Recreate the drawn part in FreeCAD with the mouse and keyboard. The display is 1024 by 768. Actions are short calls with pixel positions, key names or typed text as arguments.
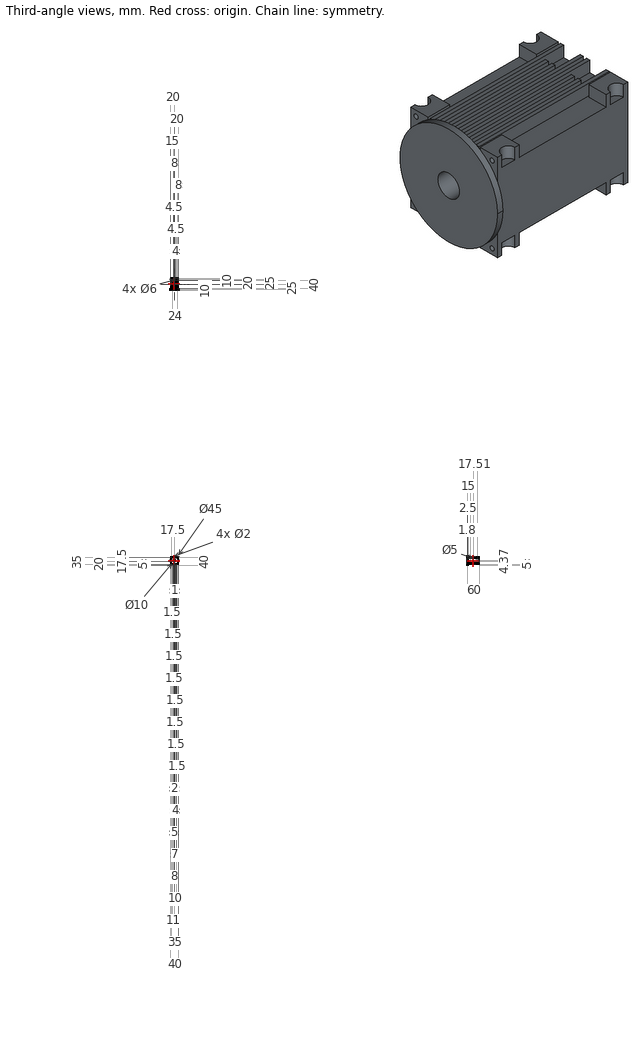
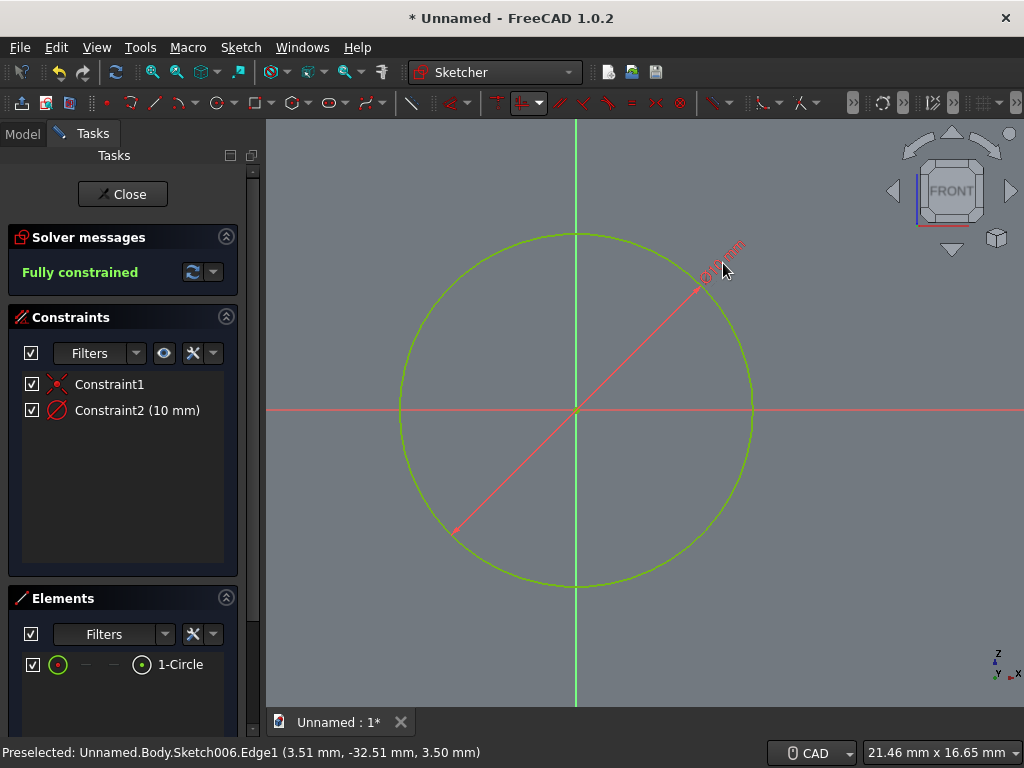
click(123, 194)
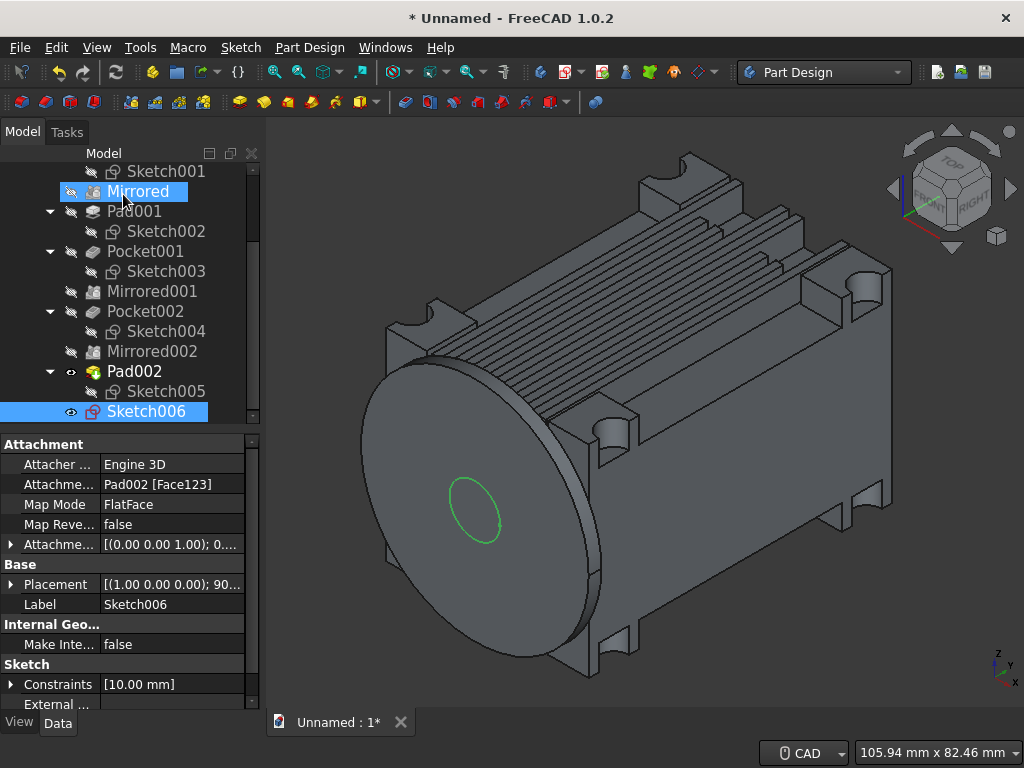
click(406, 102)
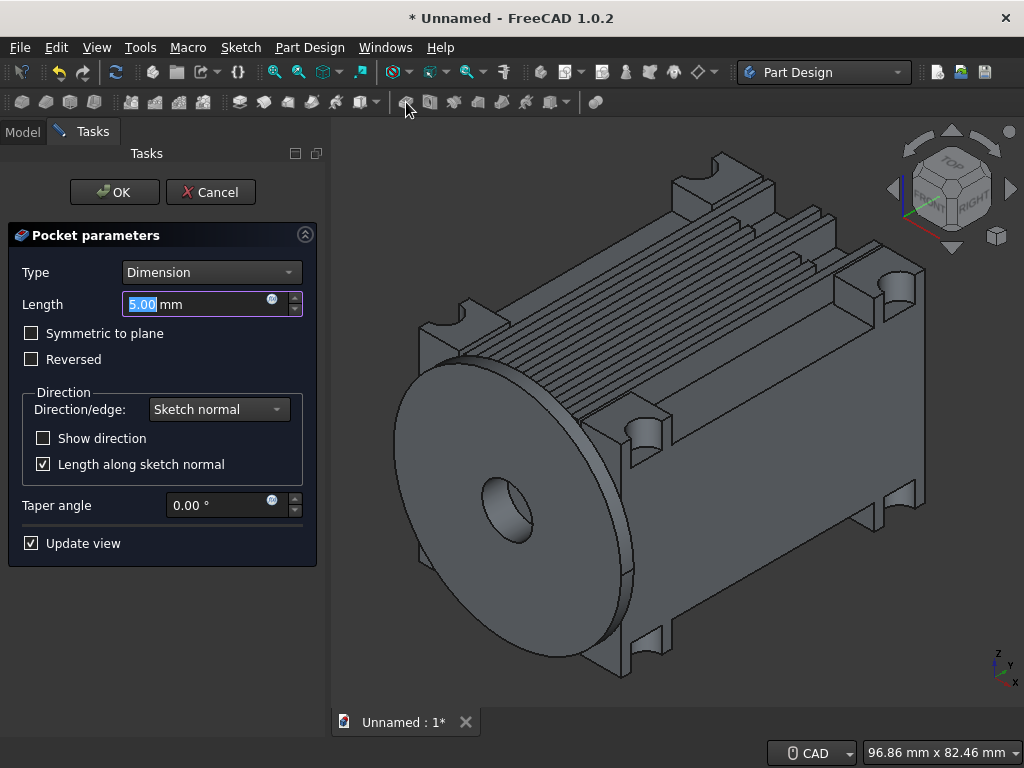
text(15)
key(Tab)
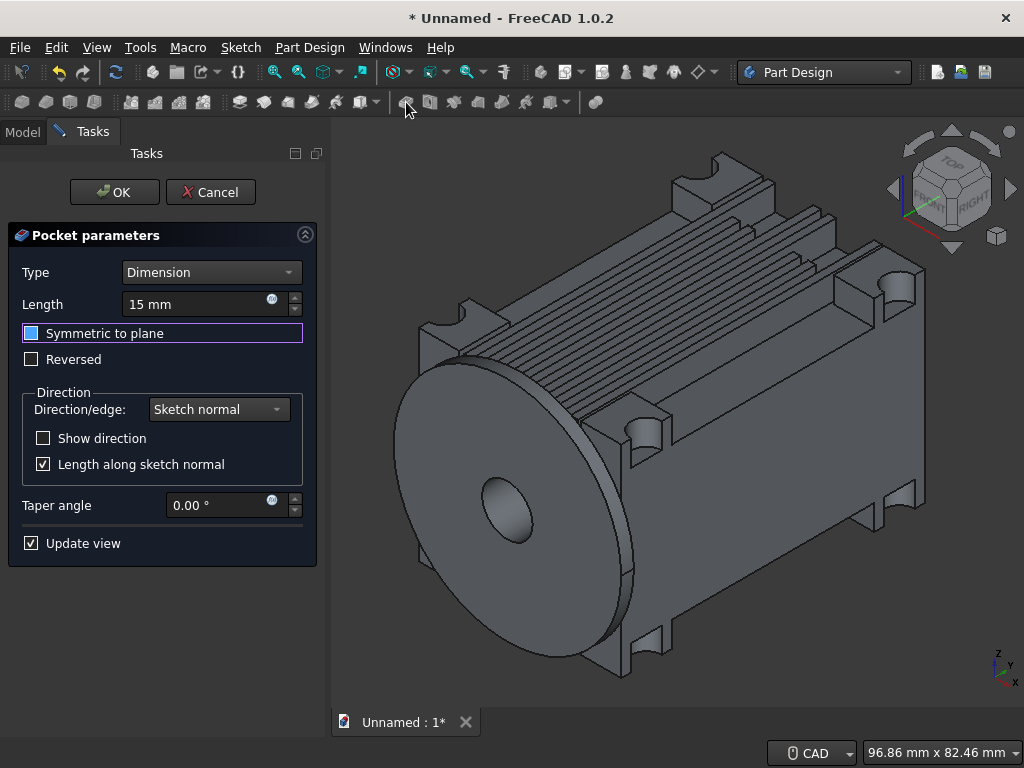
click(115, 192)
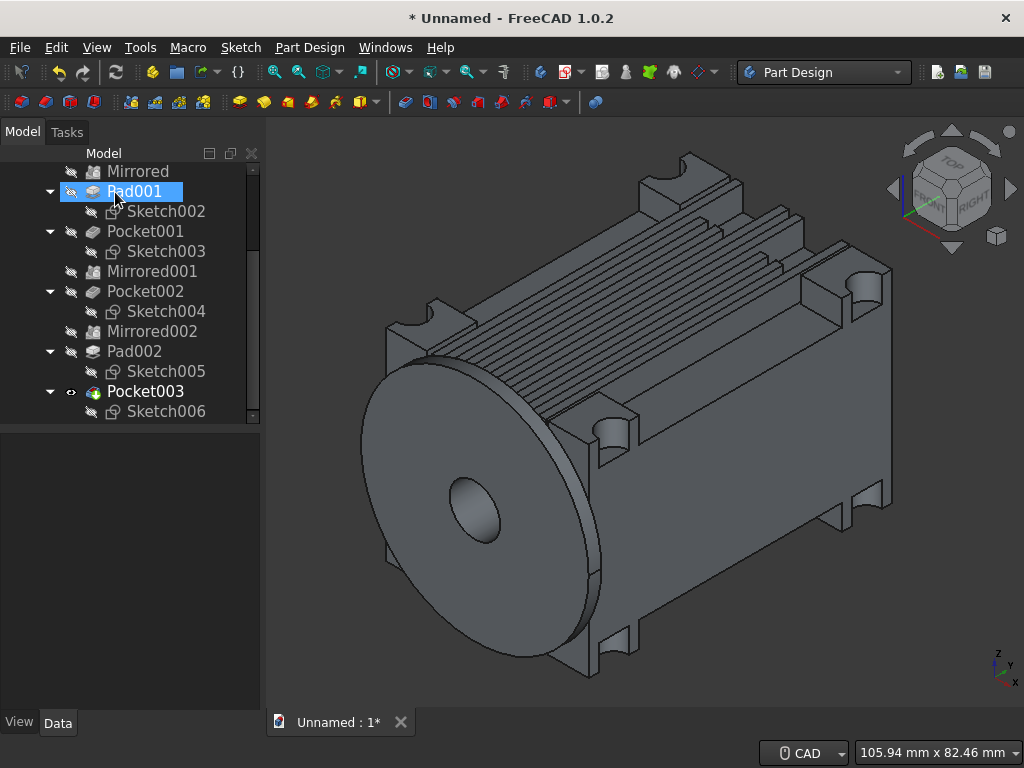
key(6)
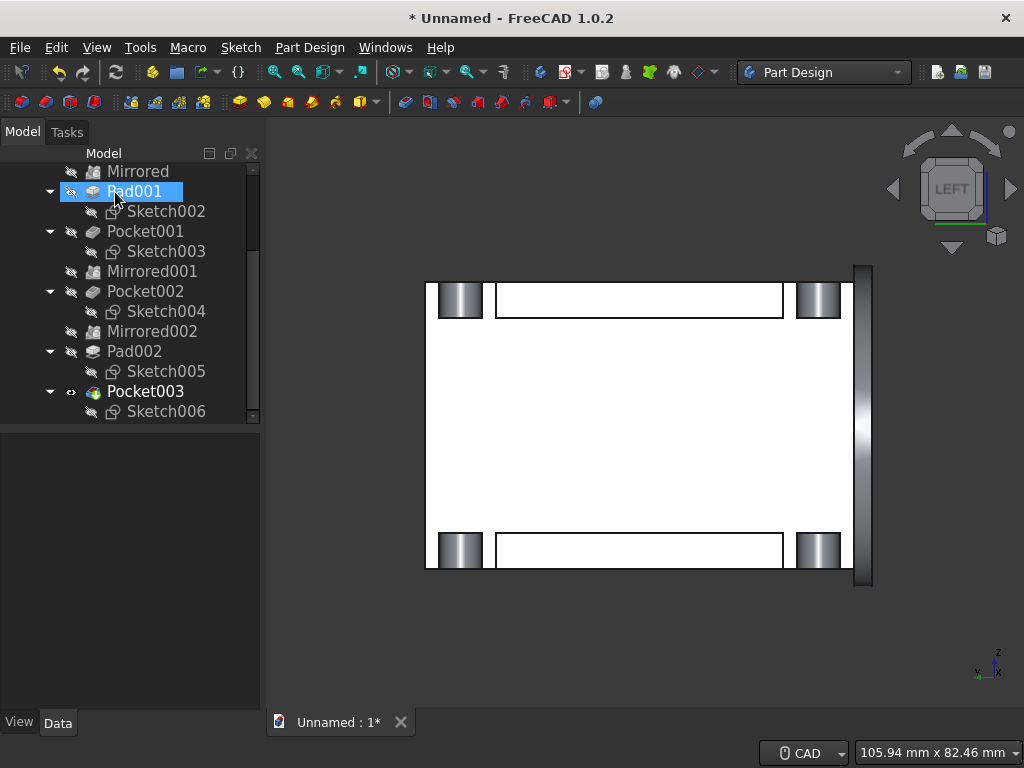
click(701, 425)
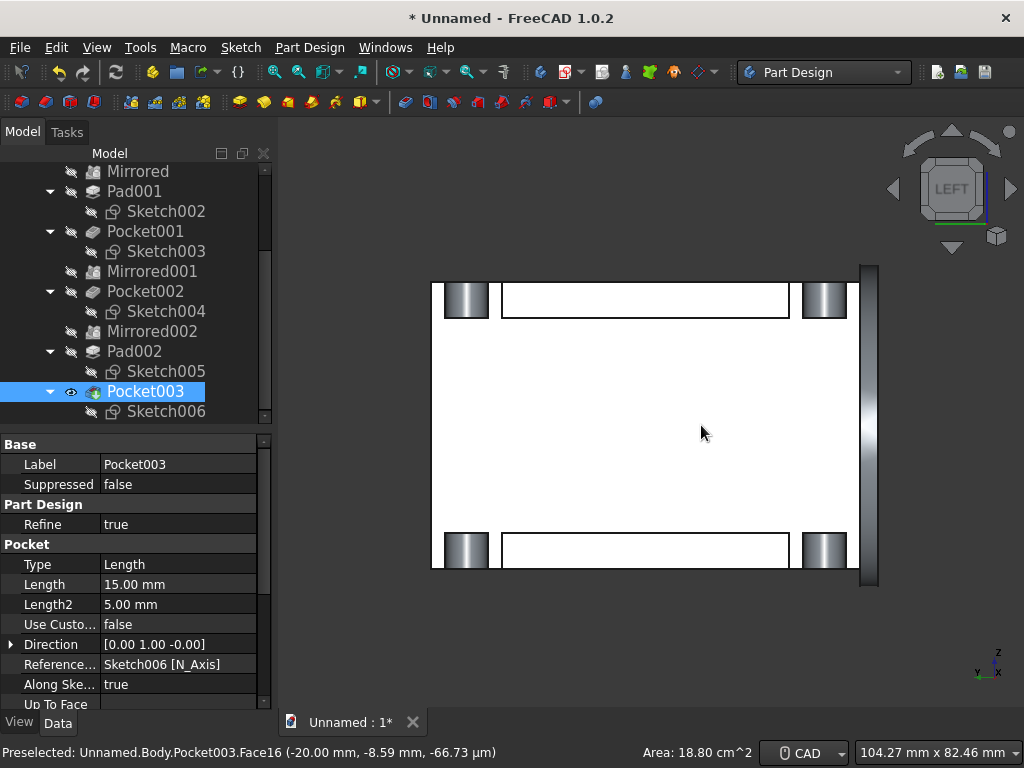
click(566, 72)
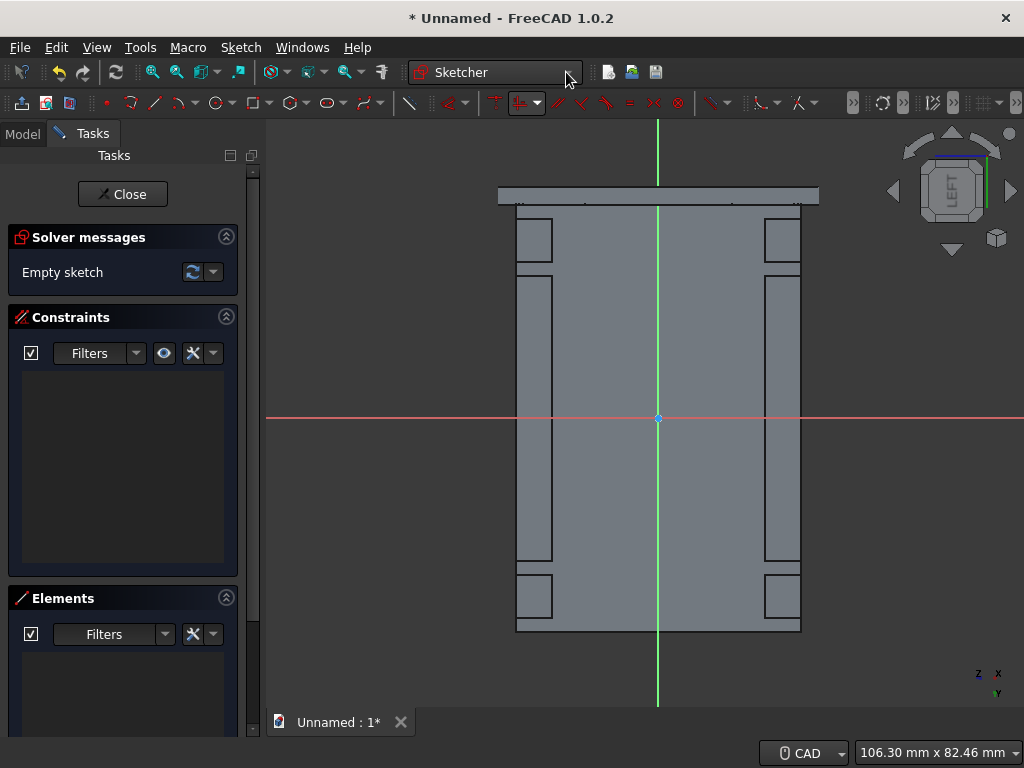
scroll(632, 556, up, 12)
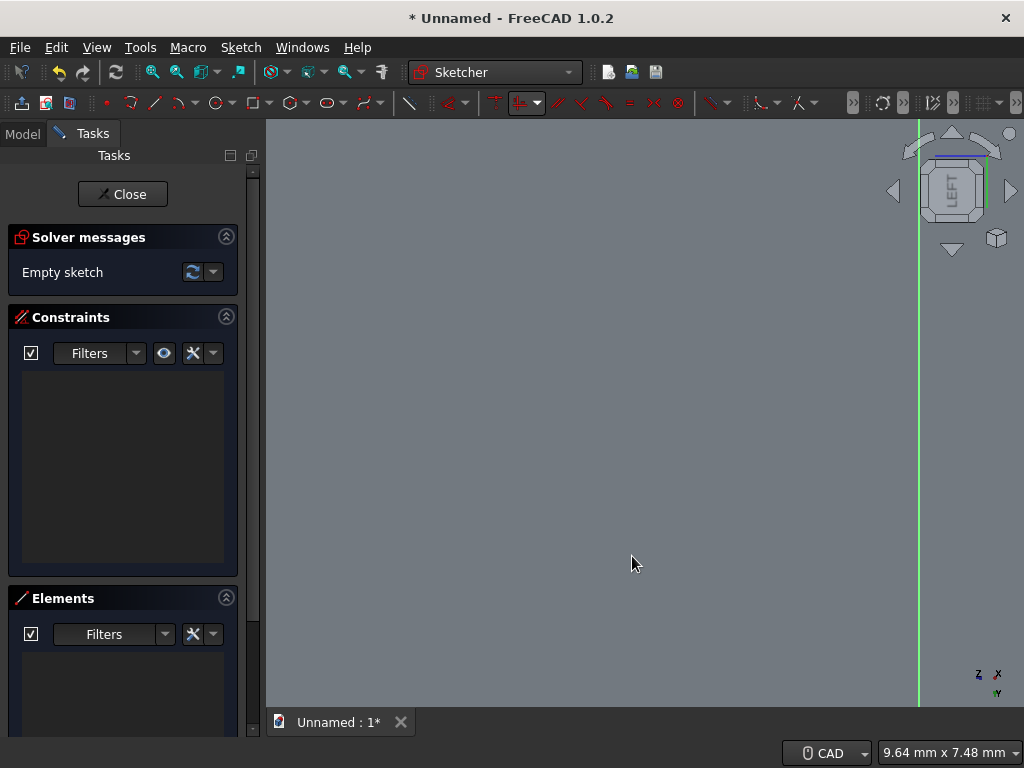
click(216, 104)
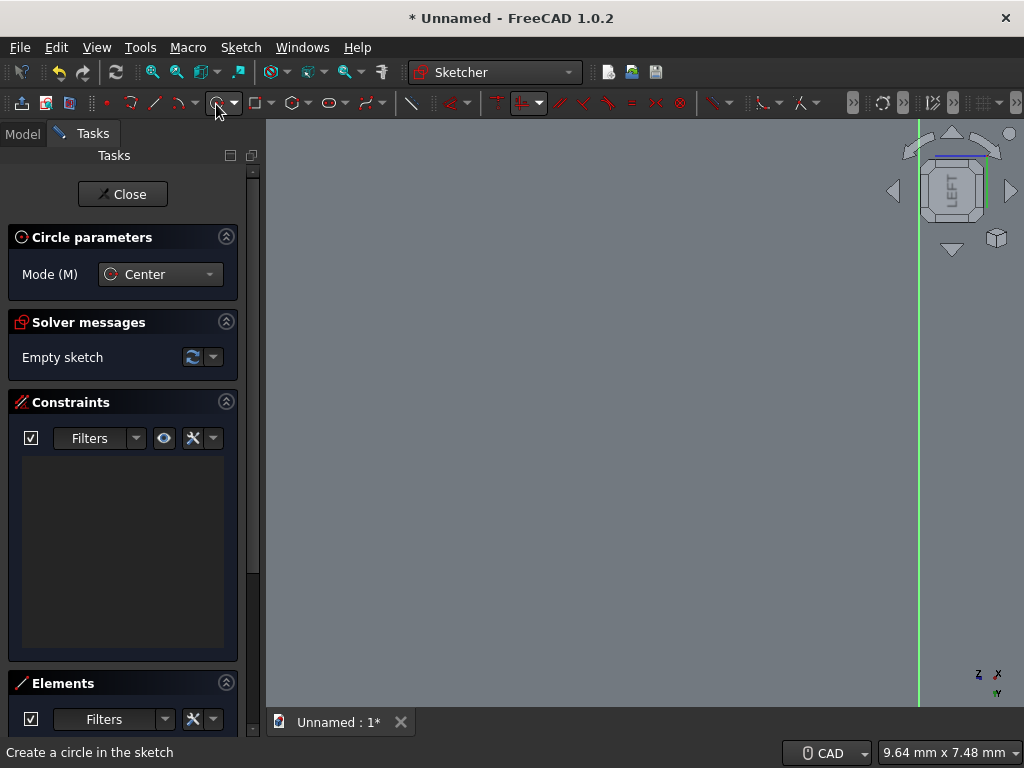
click(576, 408)
click(714, 269)
key(Escape)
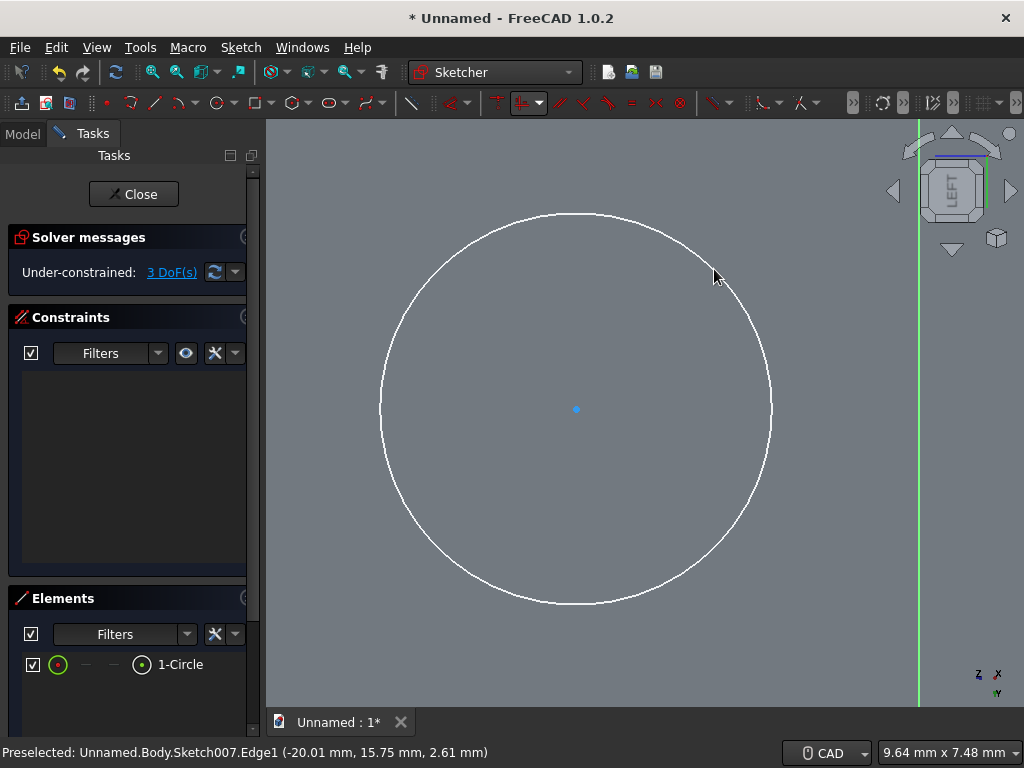
click(450, 104)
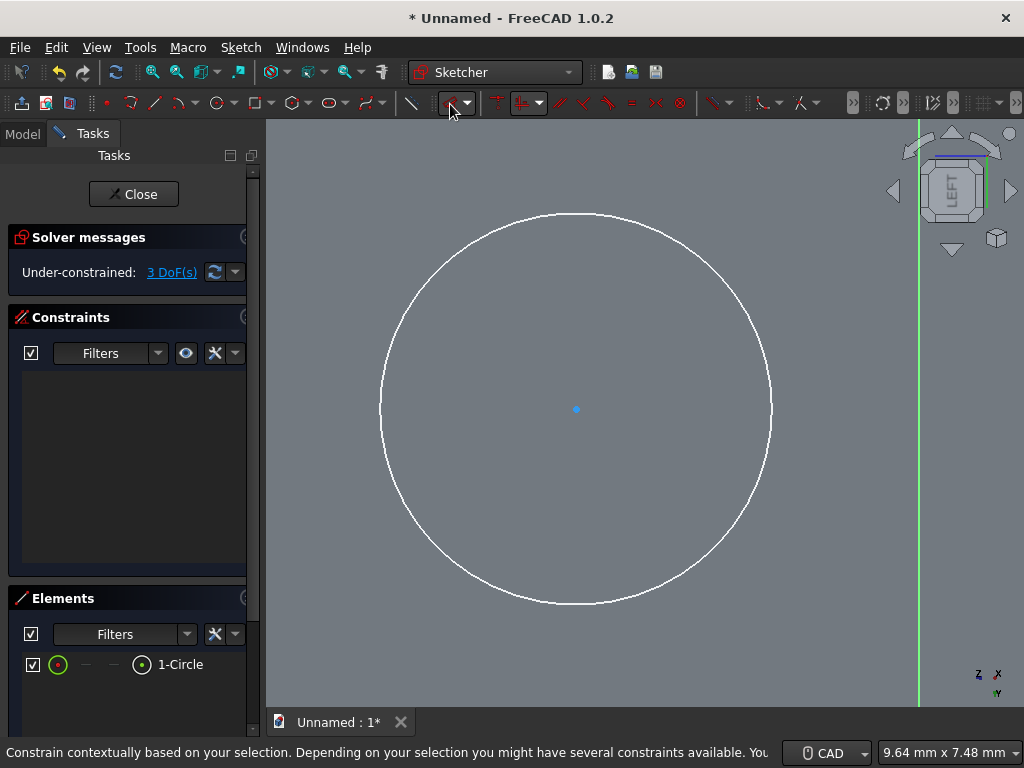
click(714, 270)
click(737, 247)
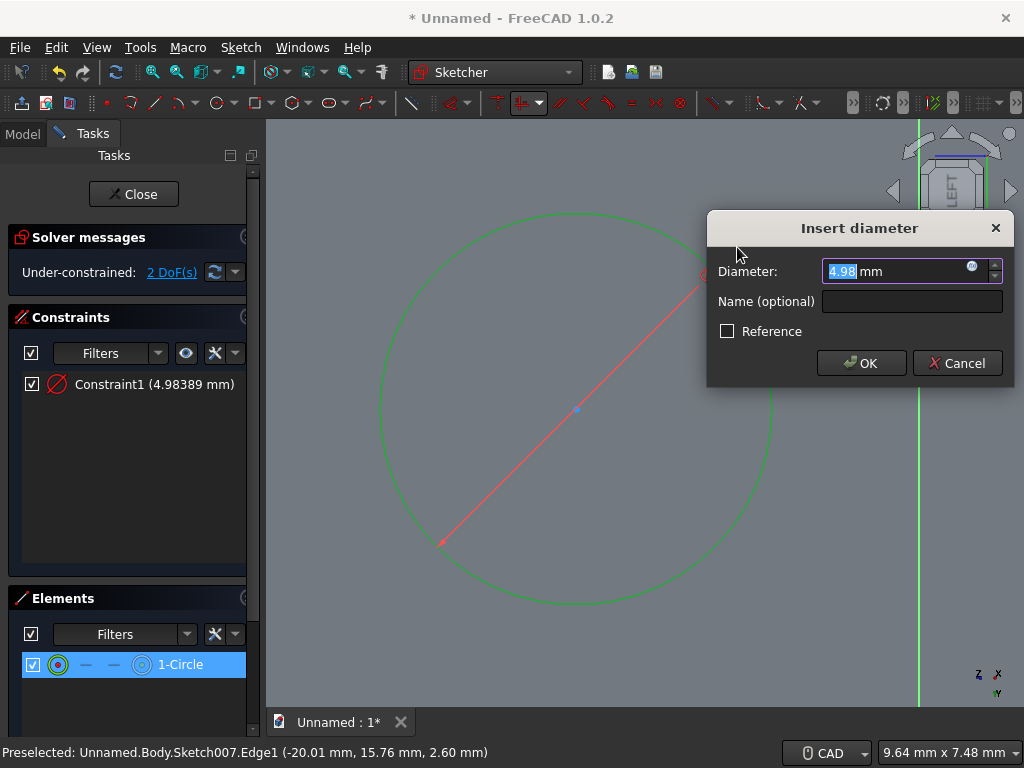
text(5)
key(Return)